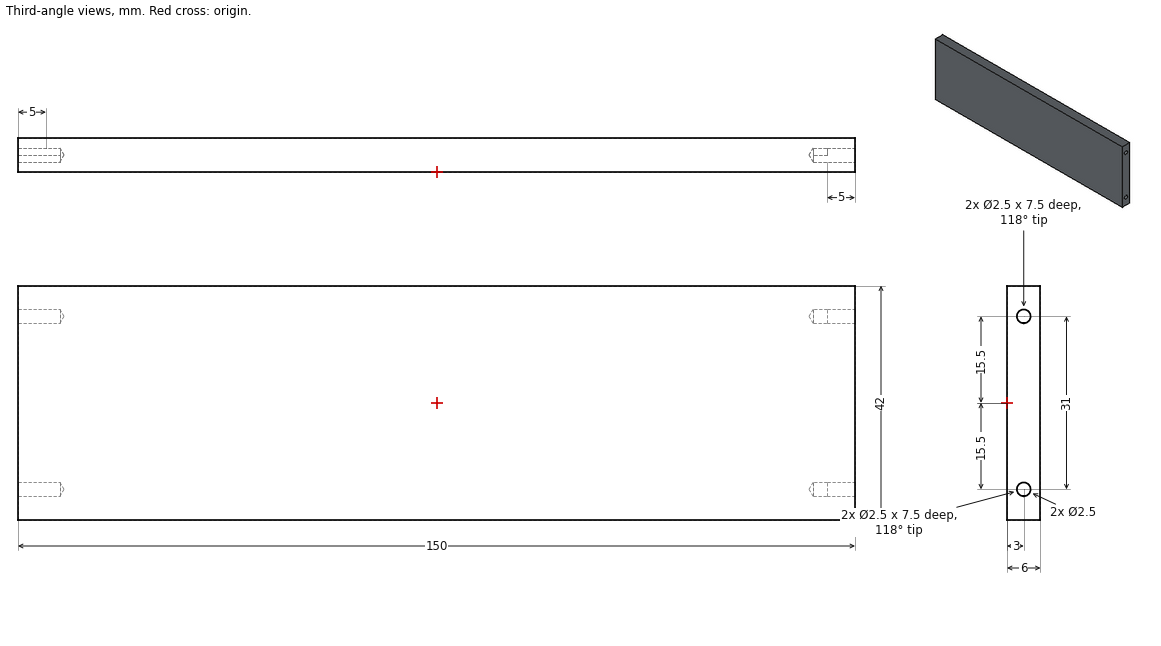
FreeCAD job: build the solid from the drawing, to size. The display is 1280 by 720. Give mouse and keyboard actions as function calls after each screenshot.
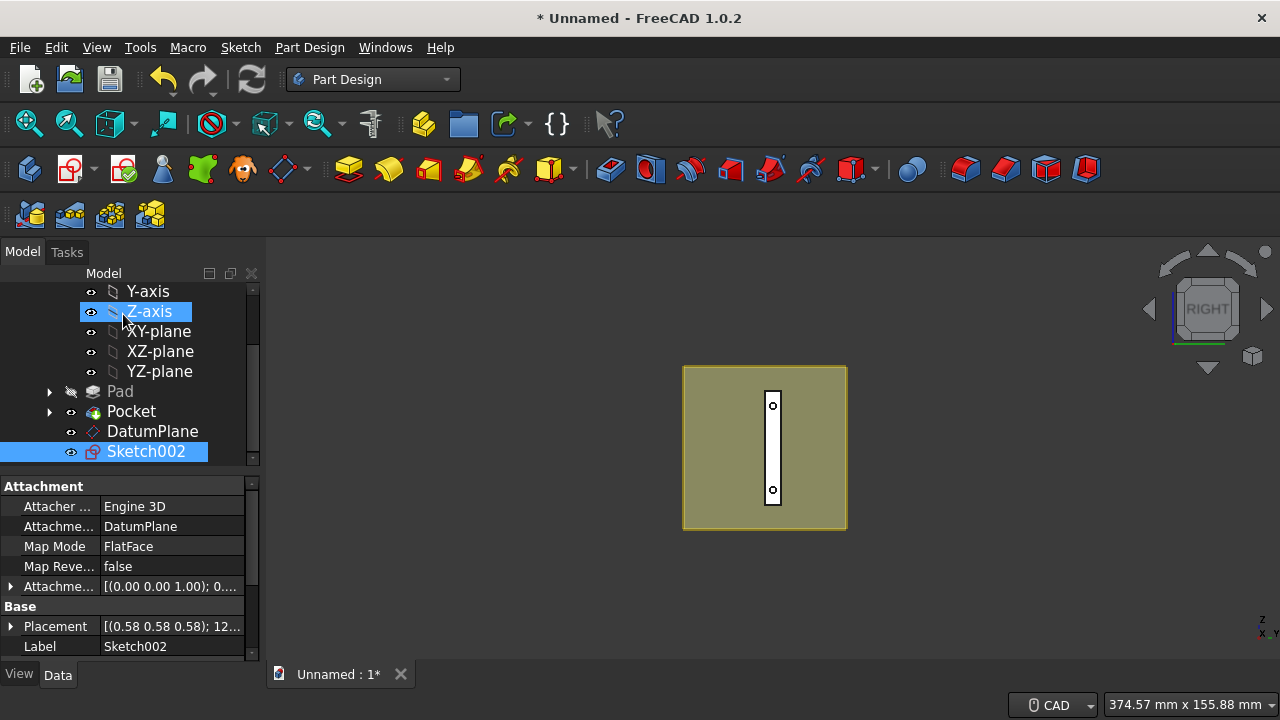
click(612, 170)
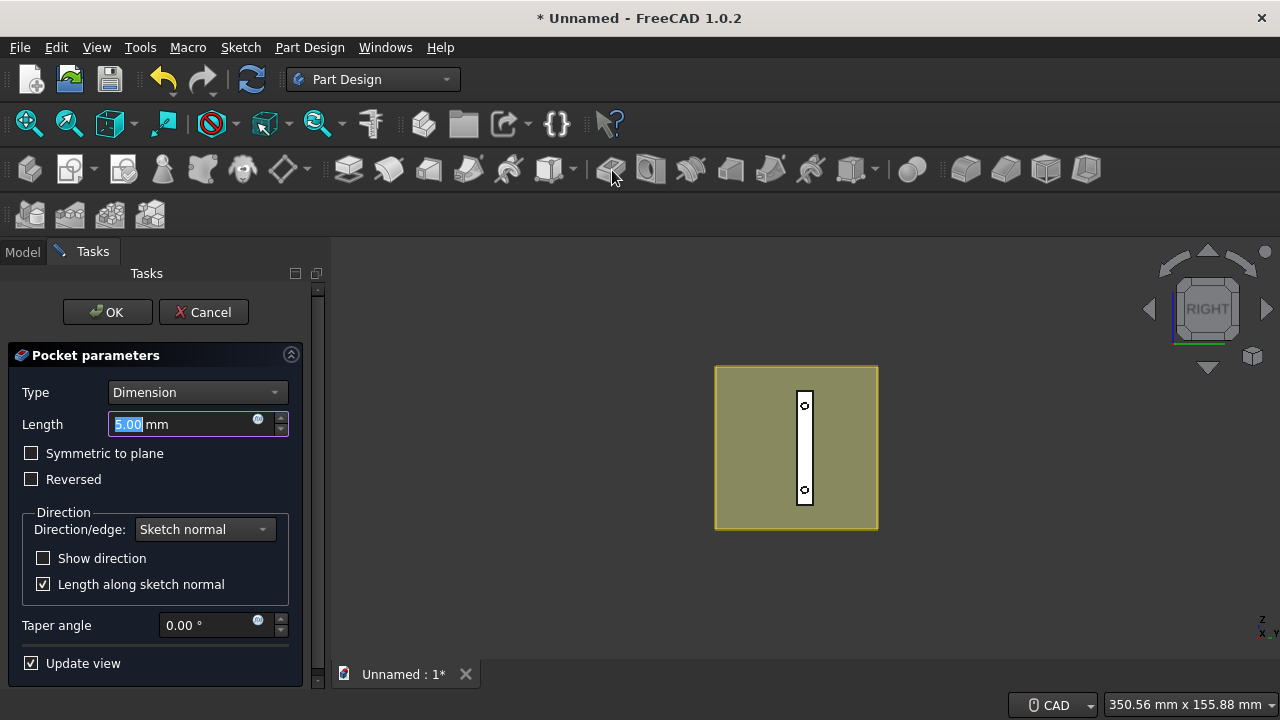
text(5)
key(Tab)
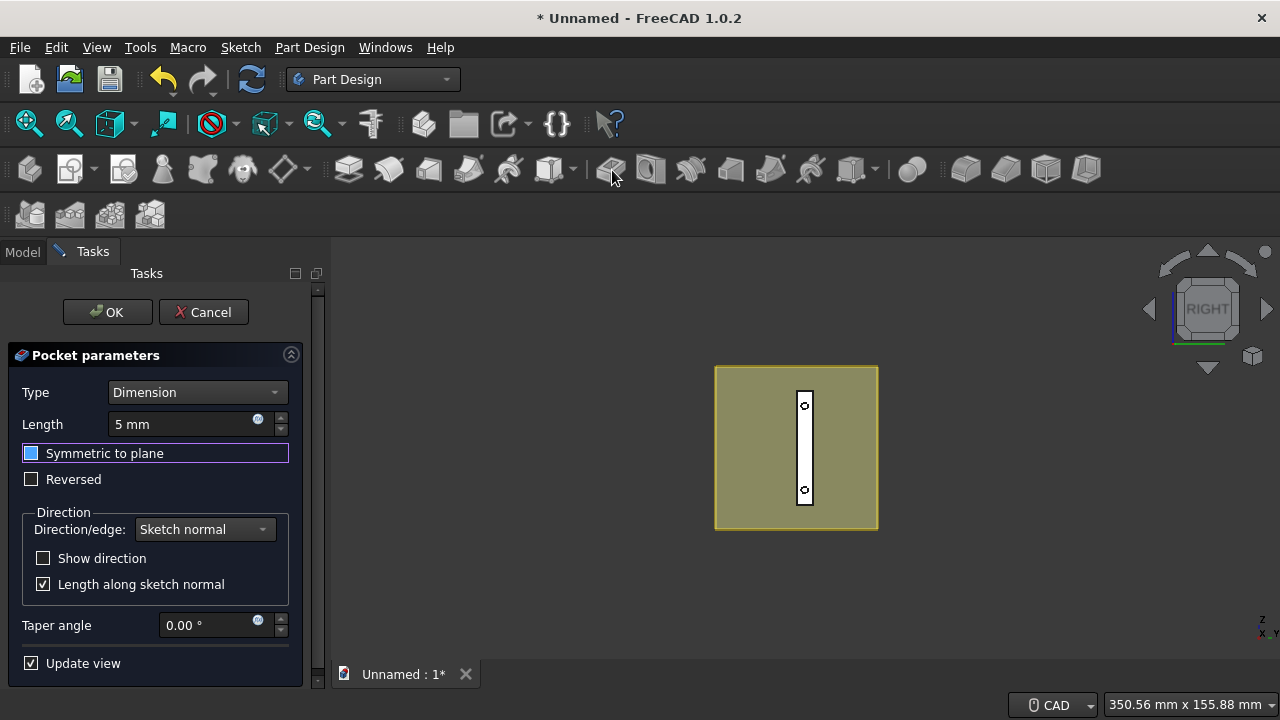
click(108, 312)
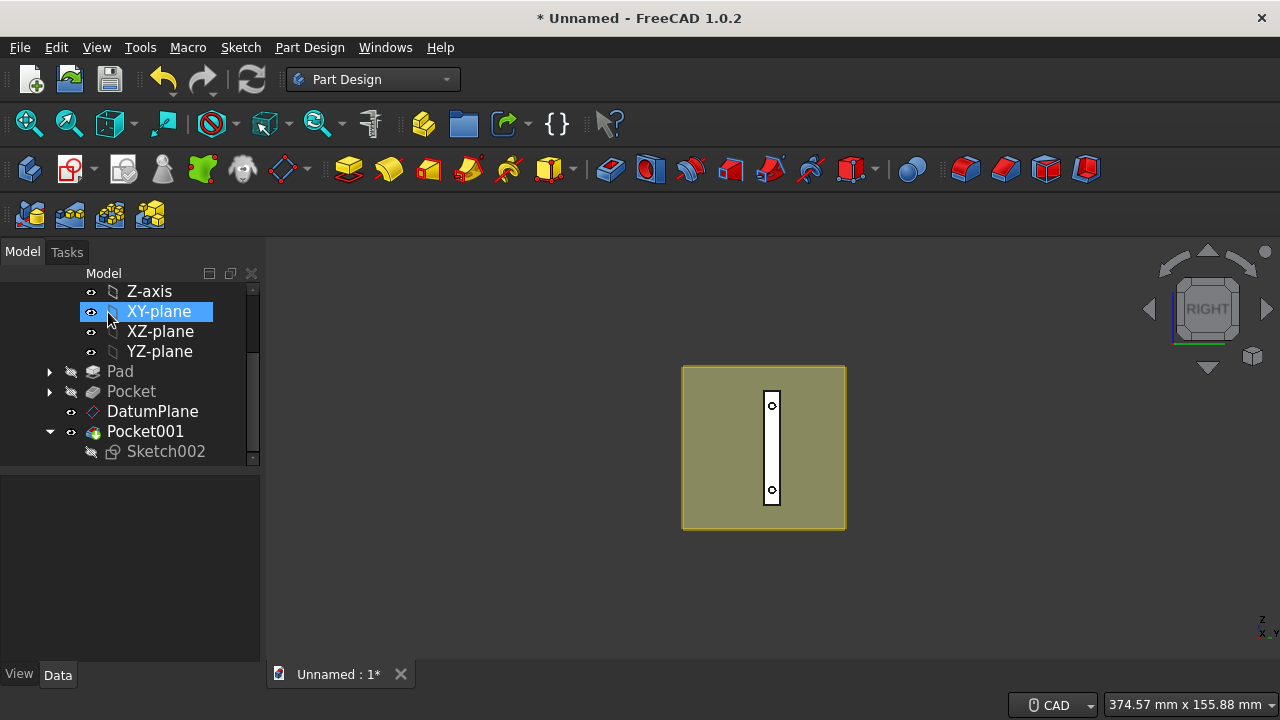
click(116, 412)
key(space)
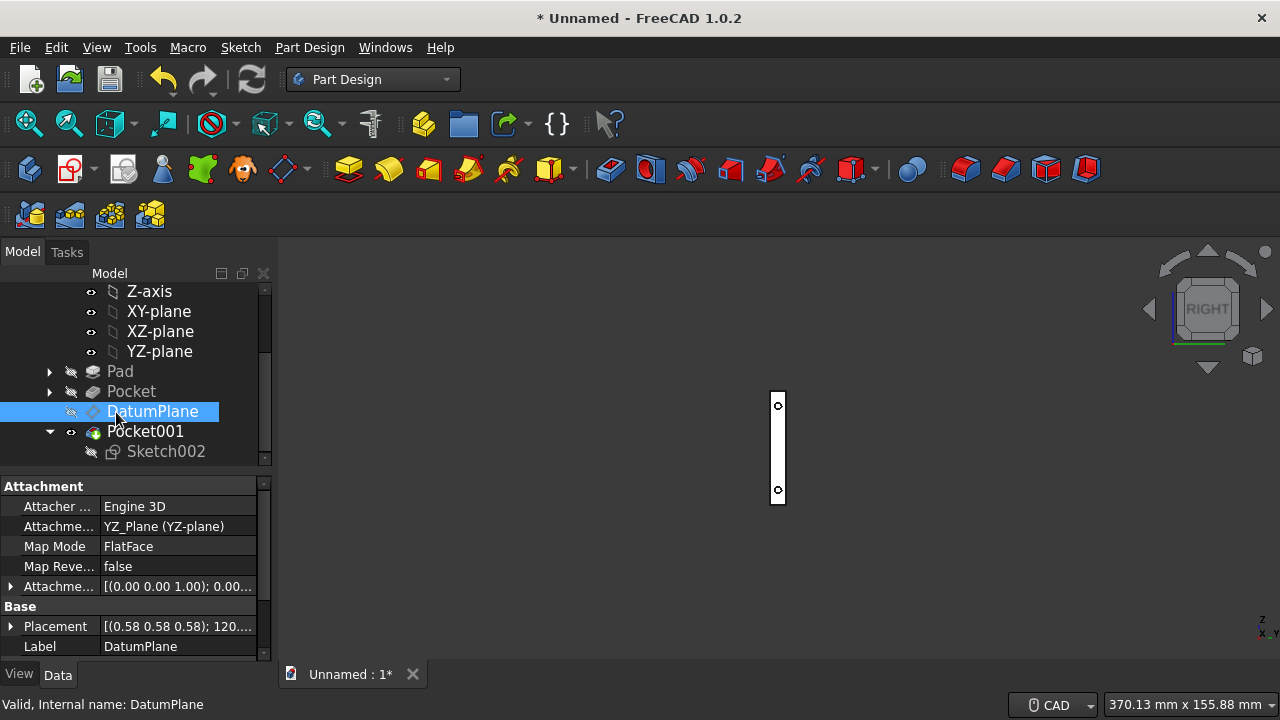
click(30, 124)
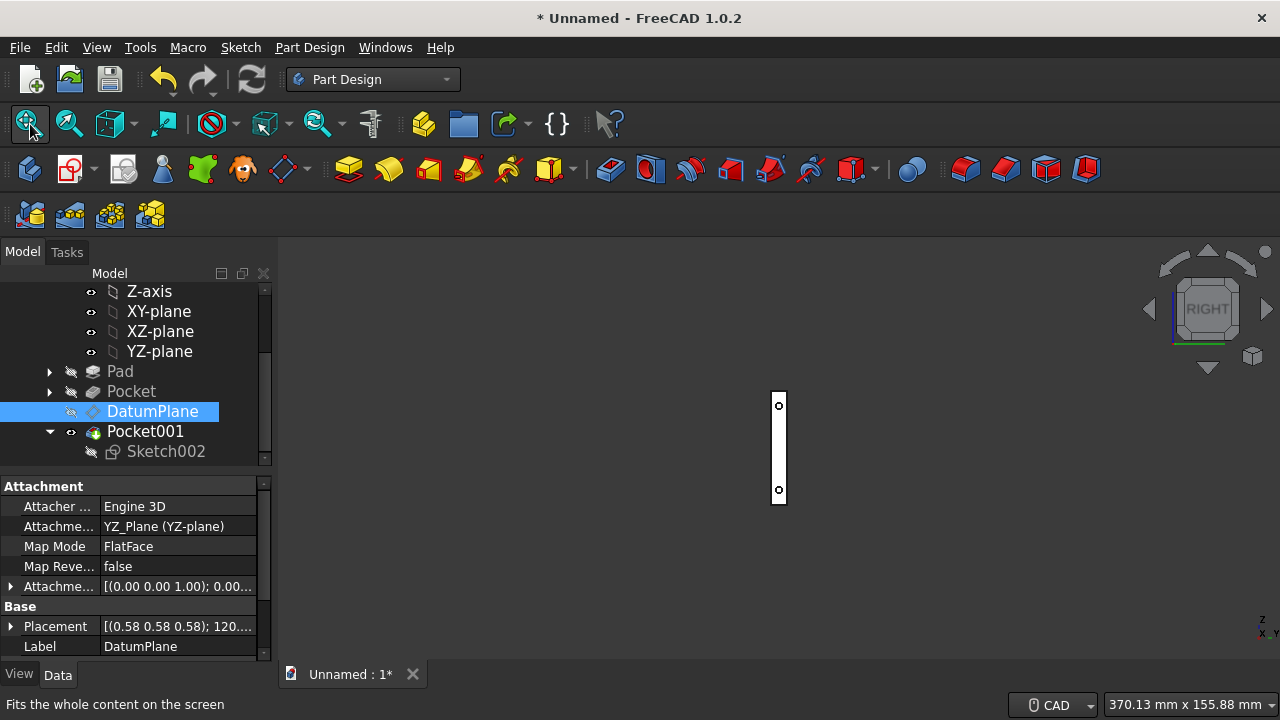
click(779, 431)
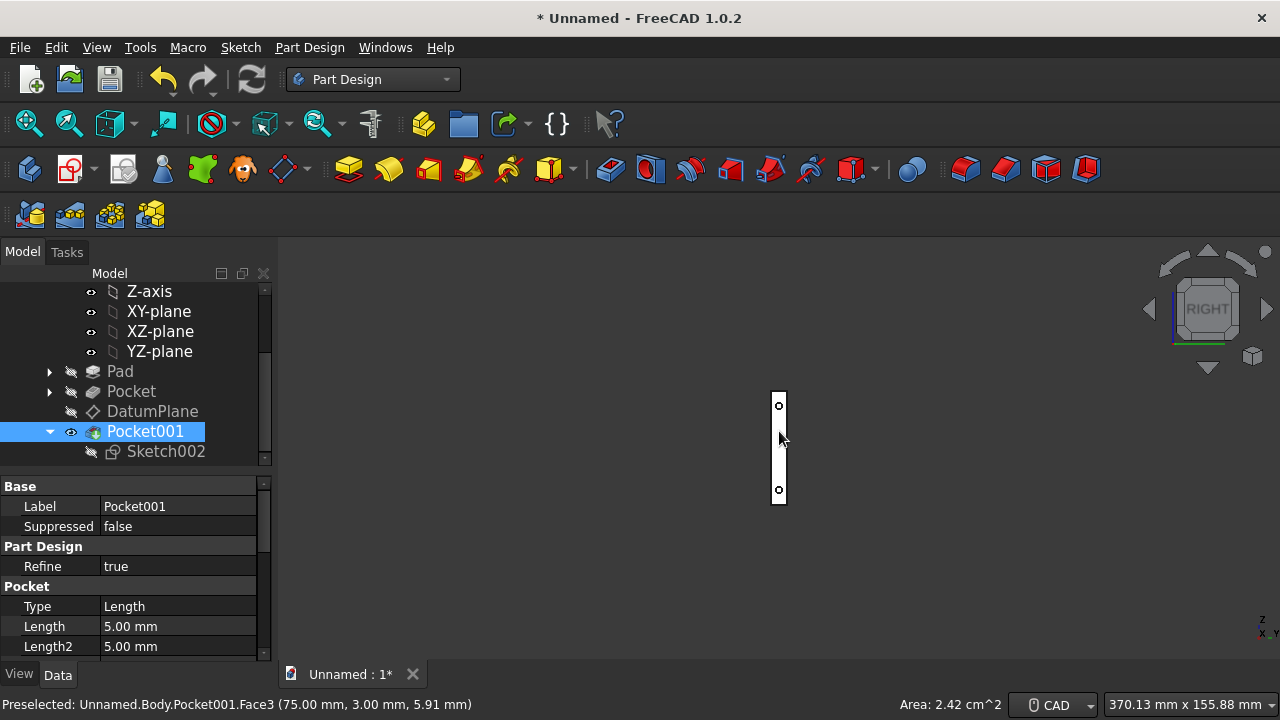
click(70, 170)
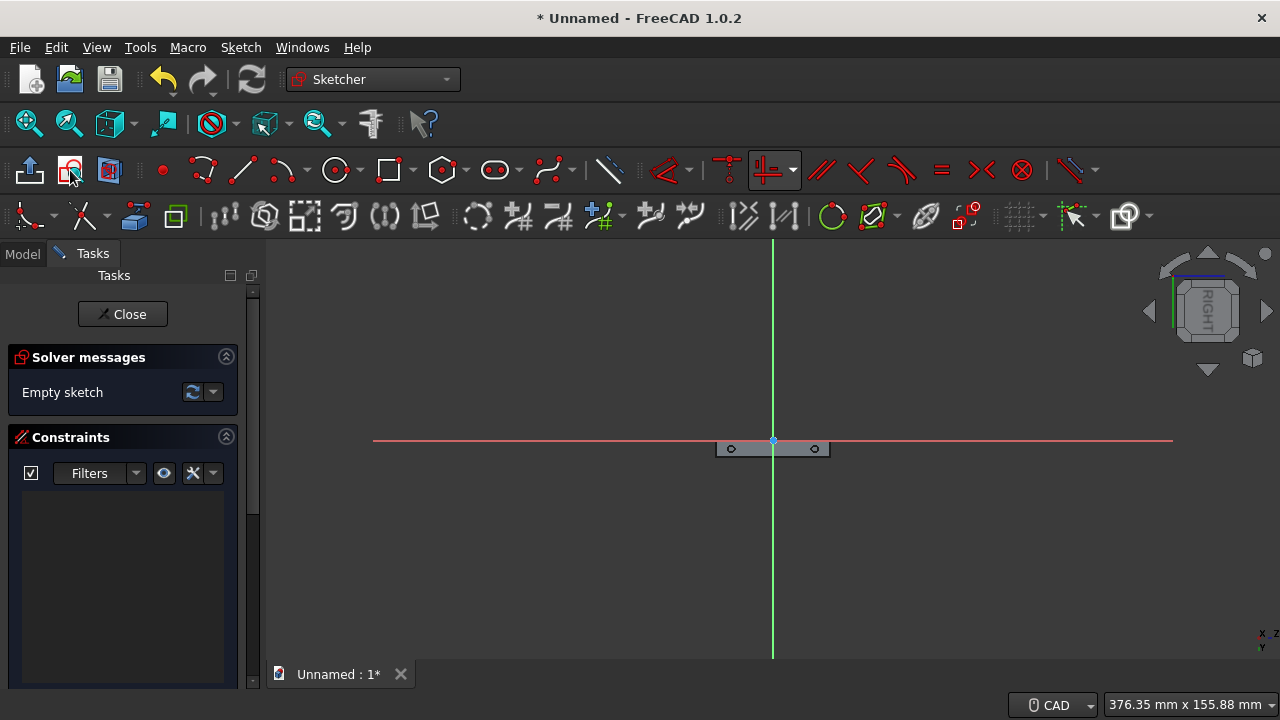
scroll(787, 446, up, 9)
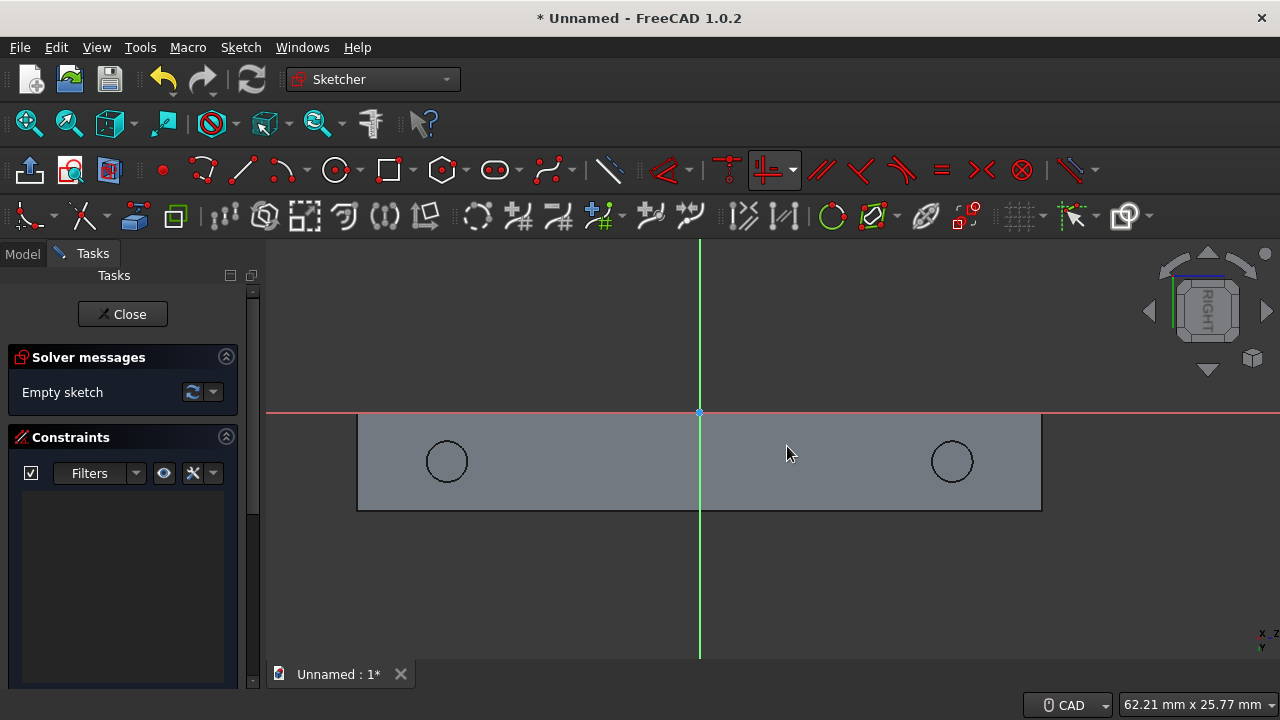
click(336, 170)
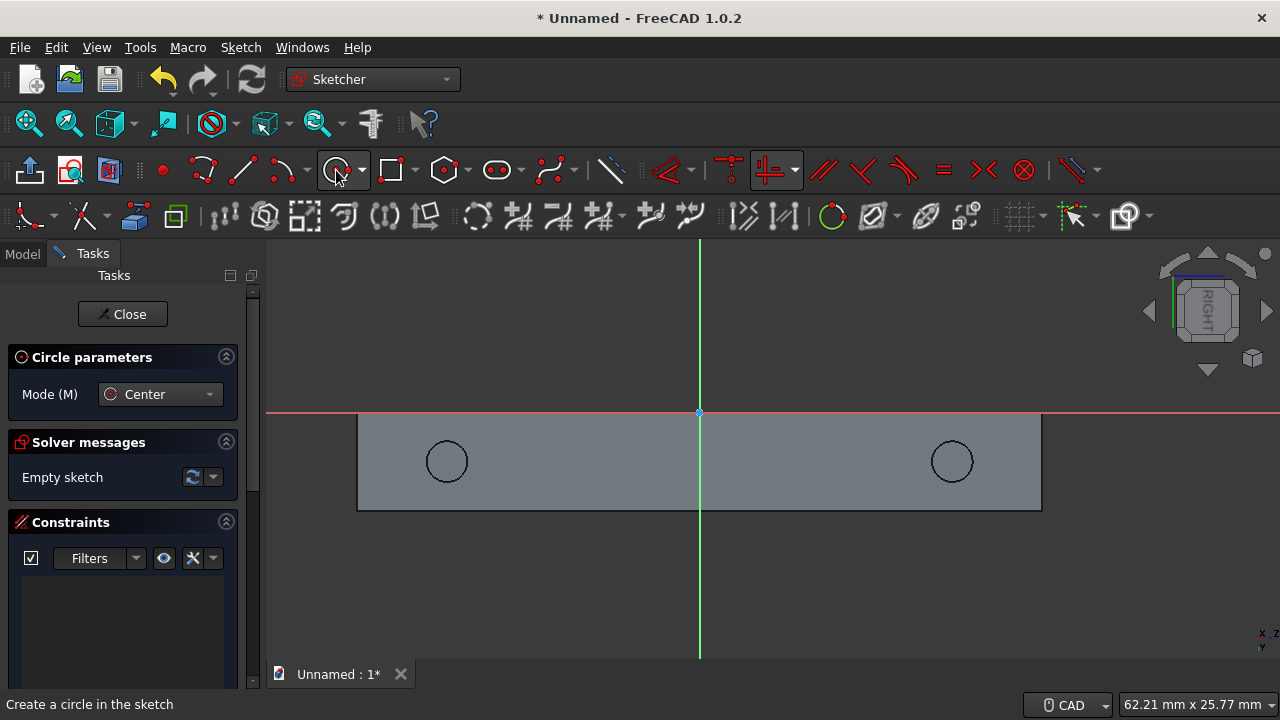
click(952, 462)
move(967, 447)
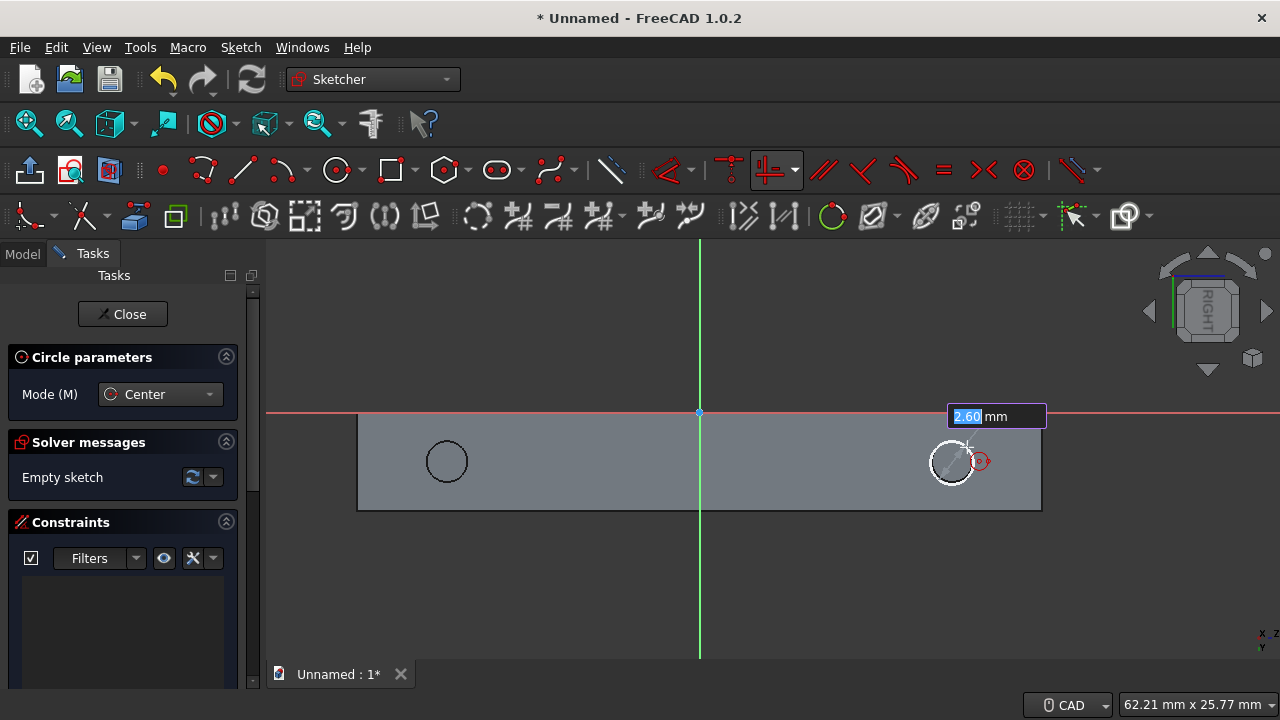
text(2.5)
key(Return)